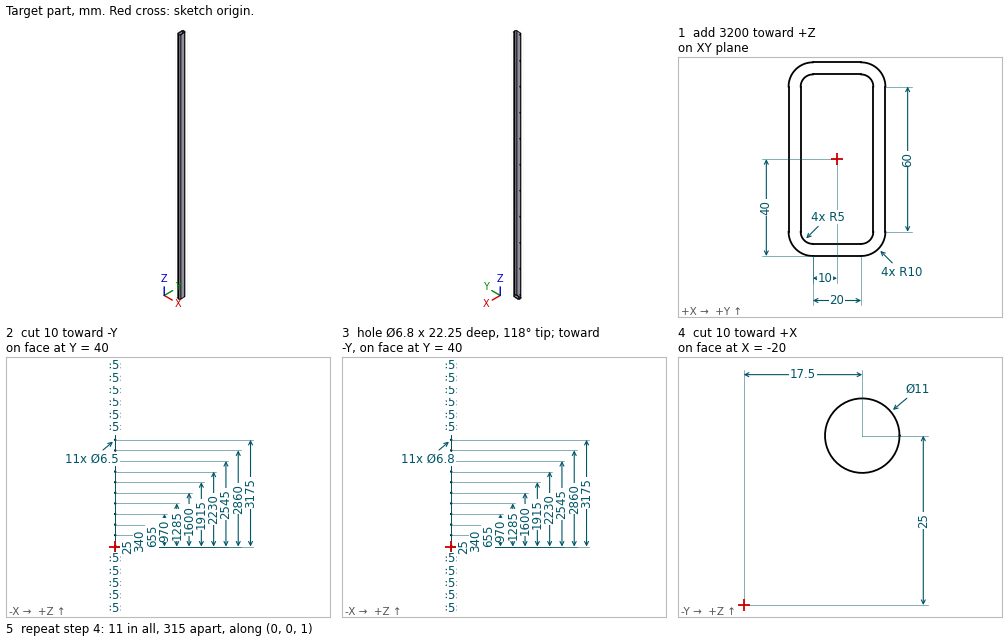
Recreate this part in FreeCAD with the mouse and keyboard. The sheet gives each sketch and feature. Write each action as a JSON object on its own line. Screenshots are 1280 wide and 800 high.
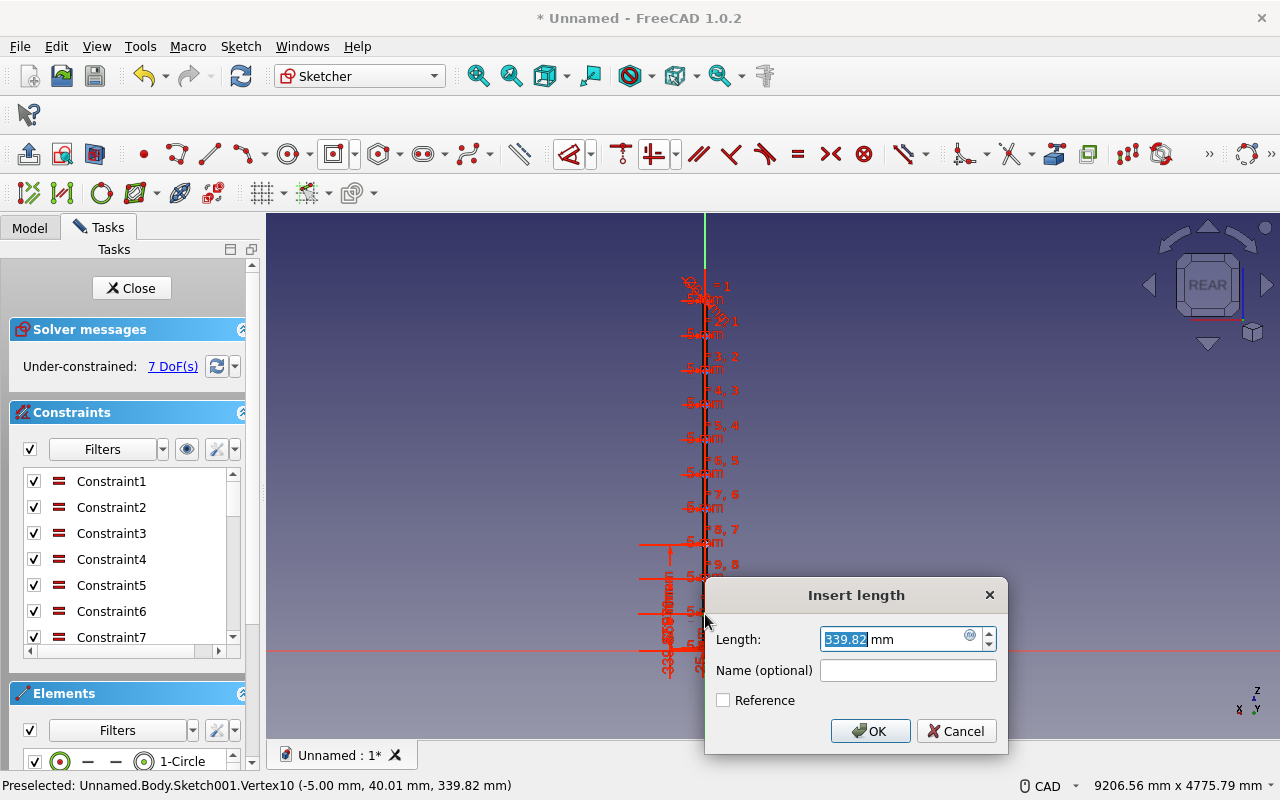
{"action": "type", "text": "340"}
{"action": "key", "text": "Return"}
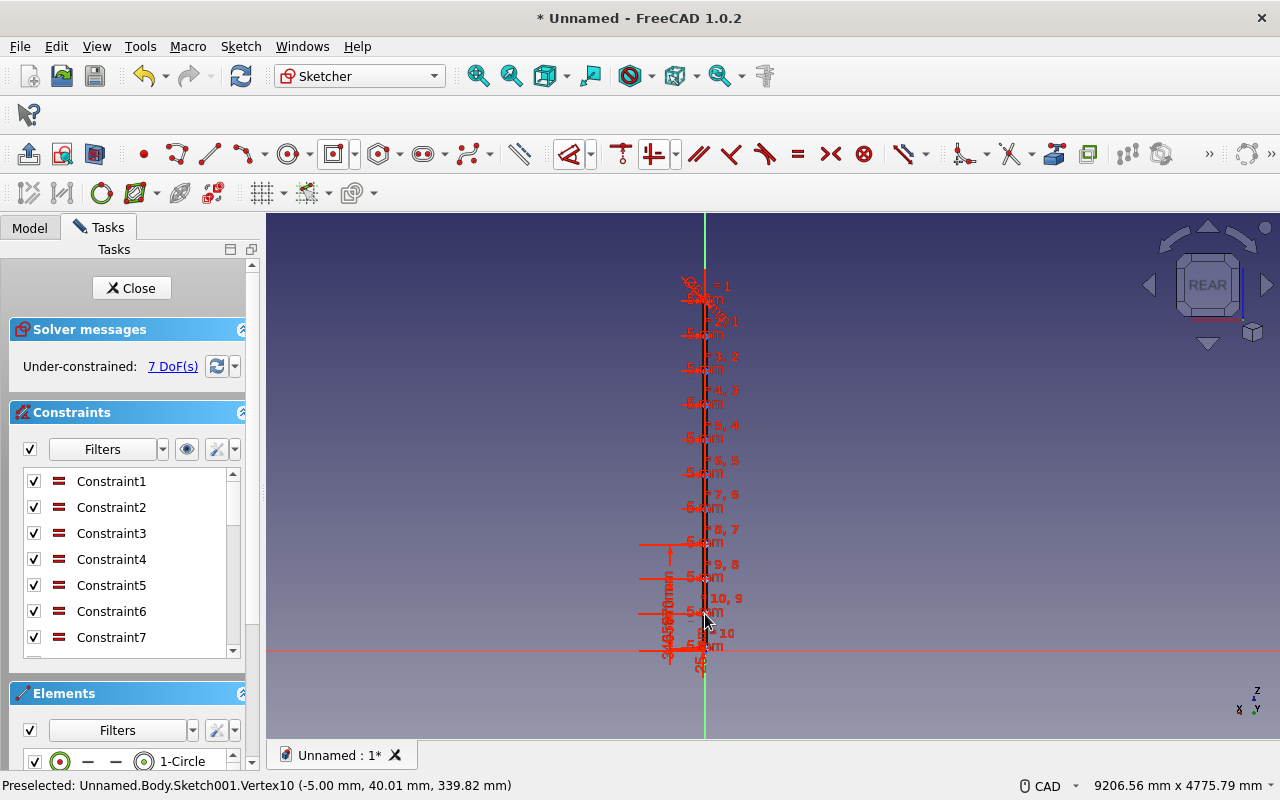
{"action": "left_click", "coordinate": [705, 302]}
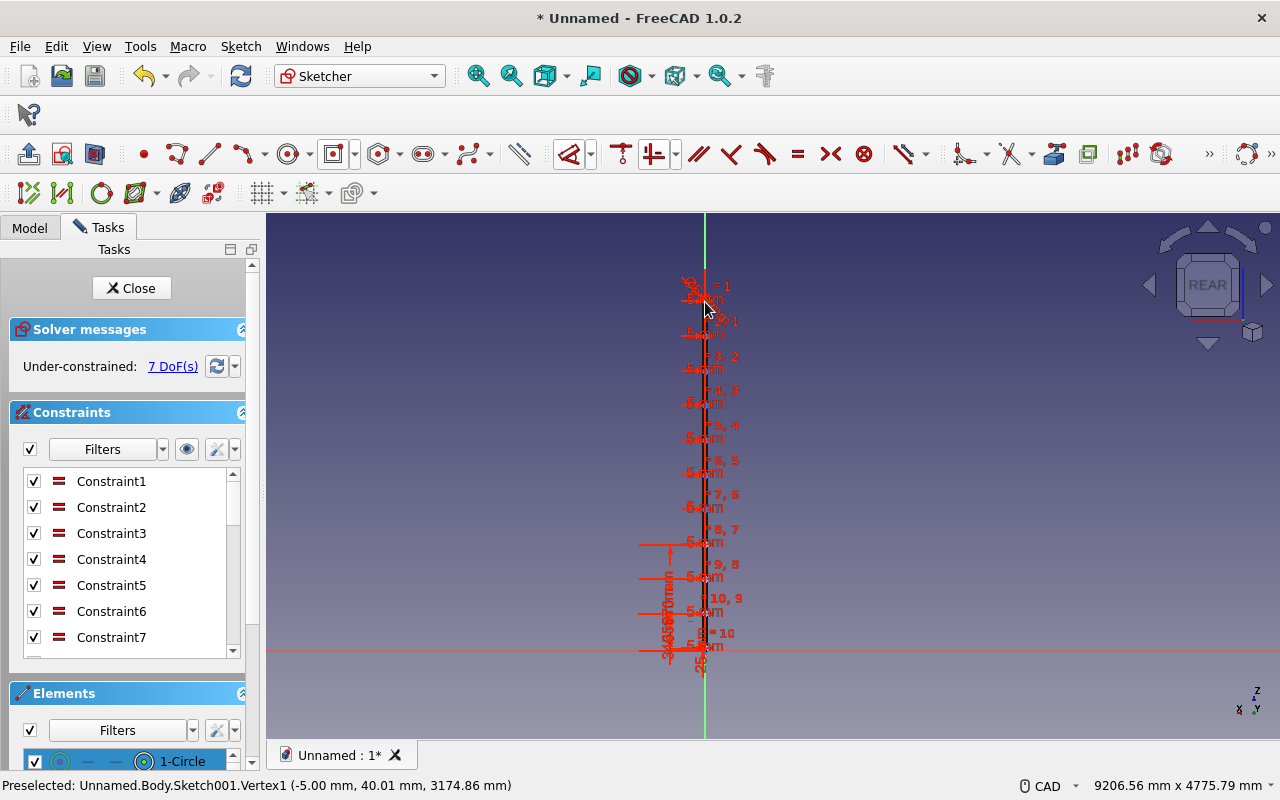
{"action": "left_click", "coordinate": [590, 154]}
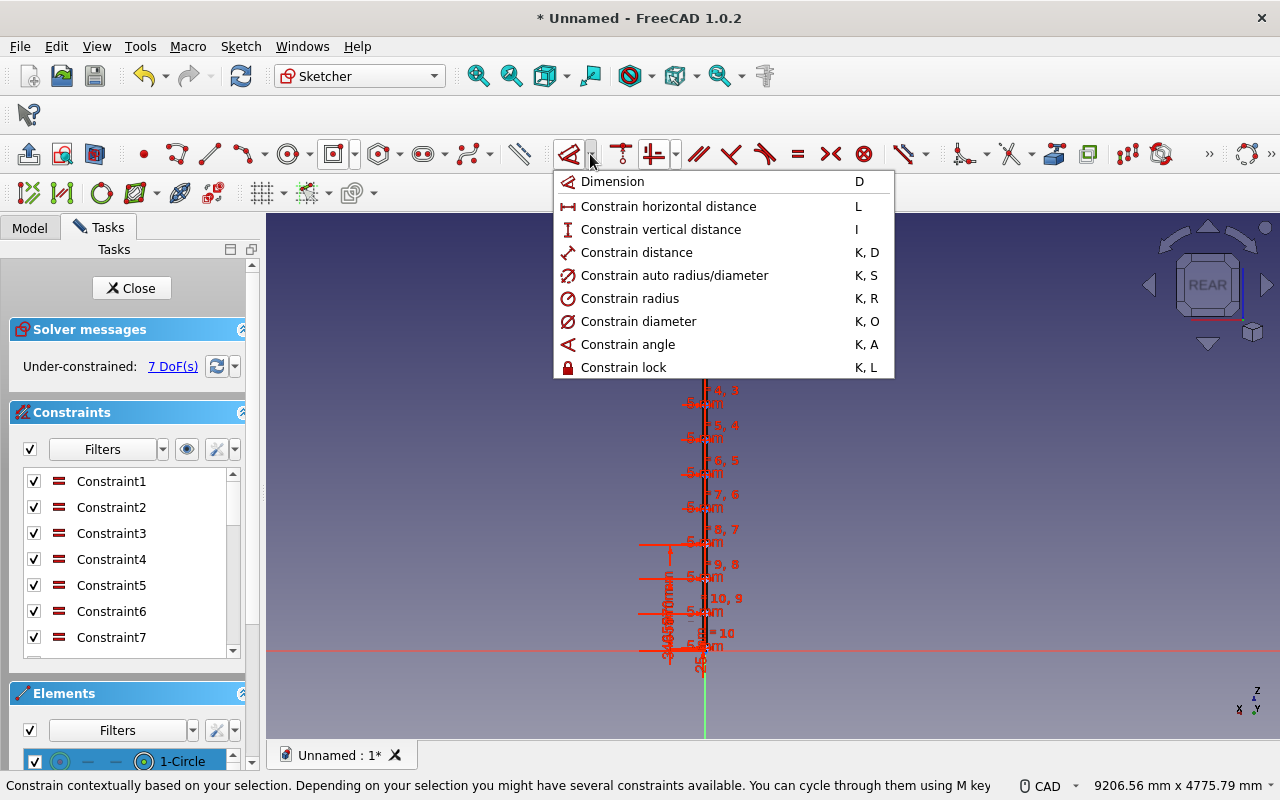
{"action": "left_click", "coordinate": [724, 230]}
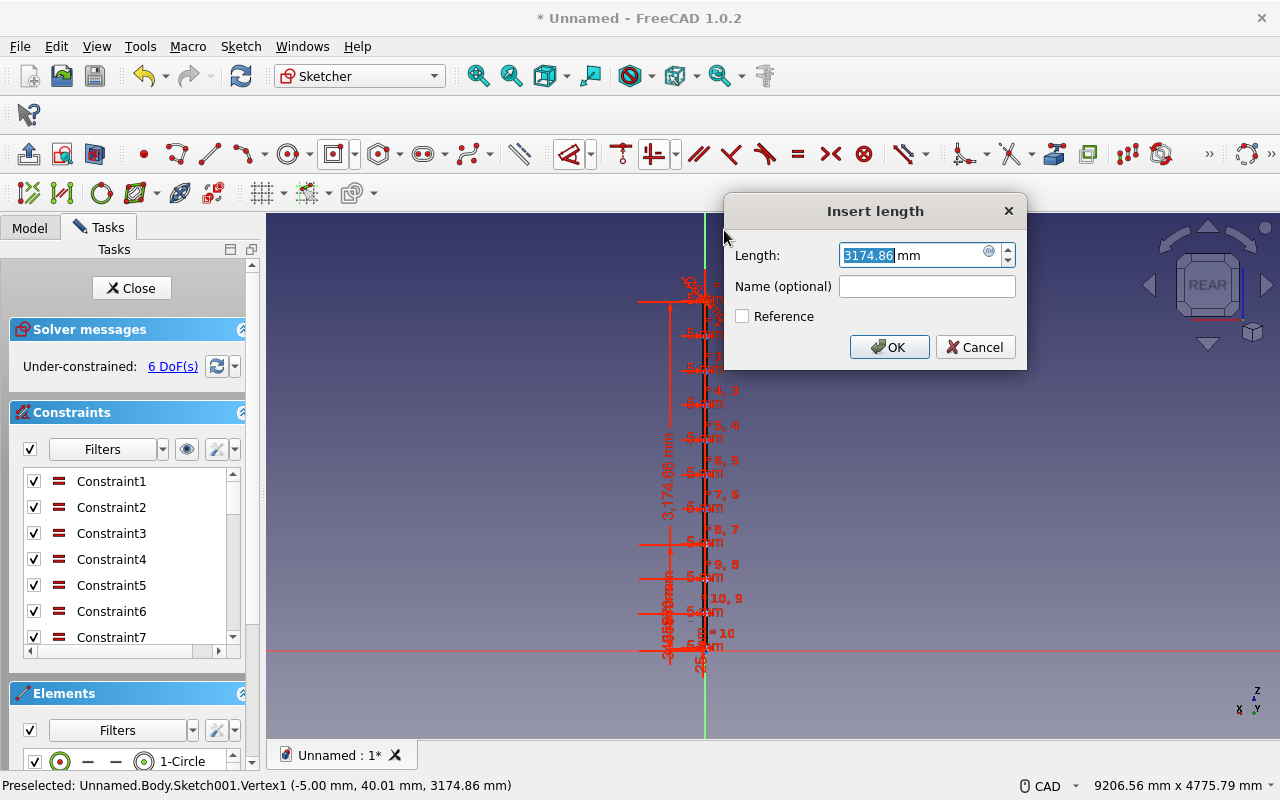
{"action": "type", "text": "3175"}
{"action": "key", "text": "Return"}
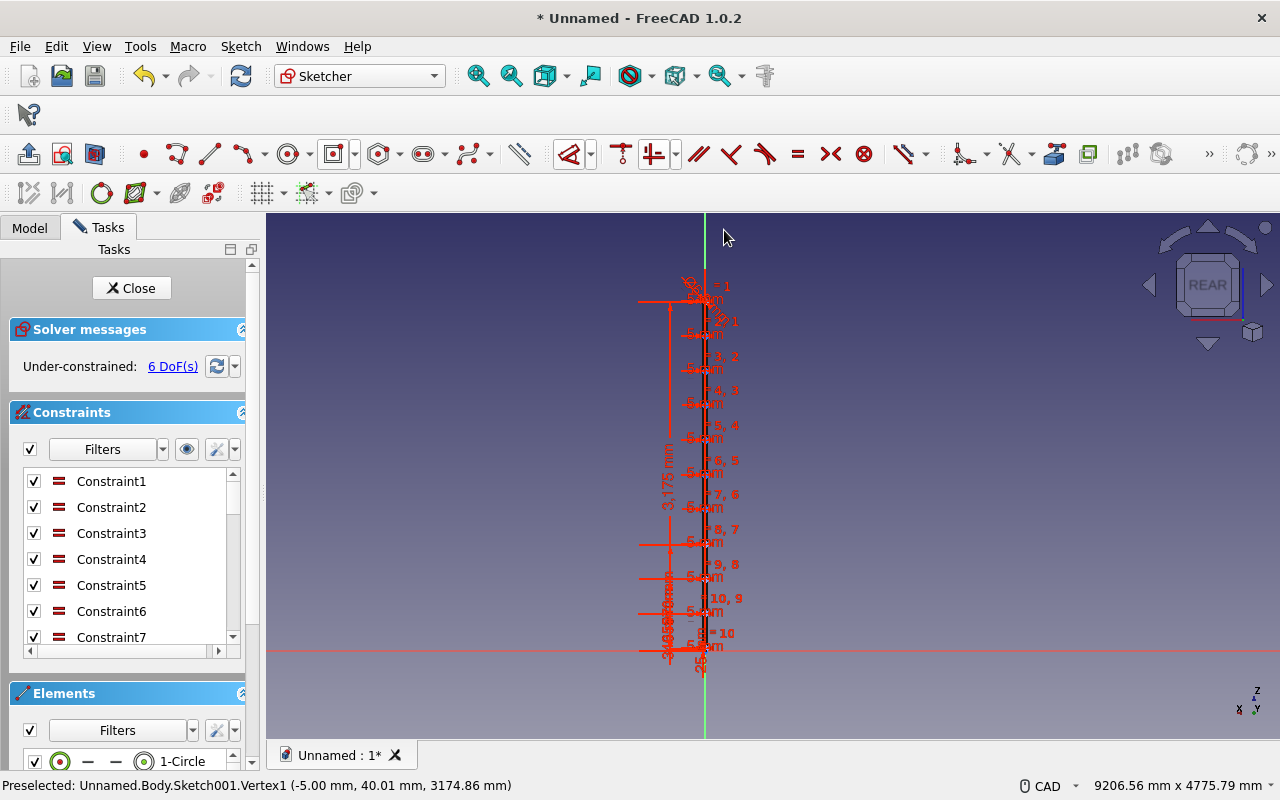
{"action": "left_click", "coordinate": [705, 336]}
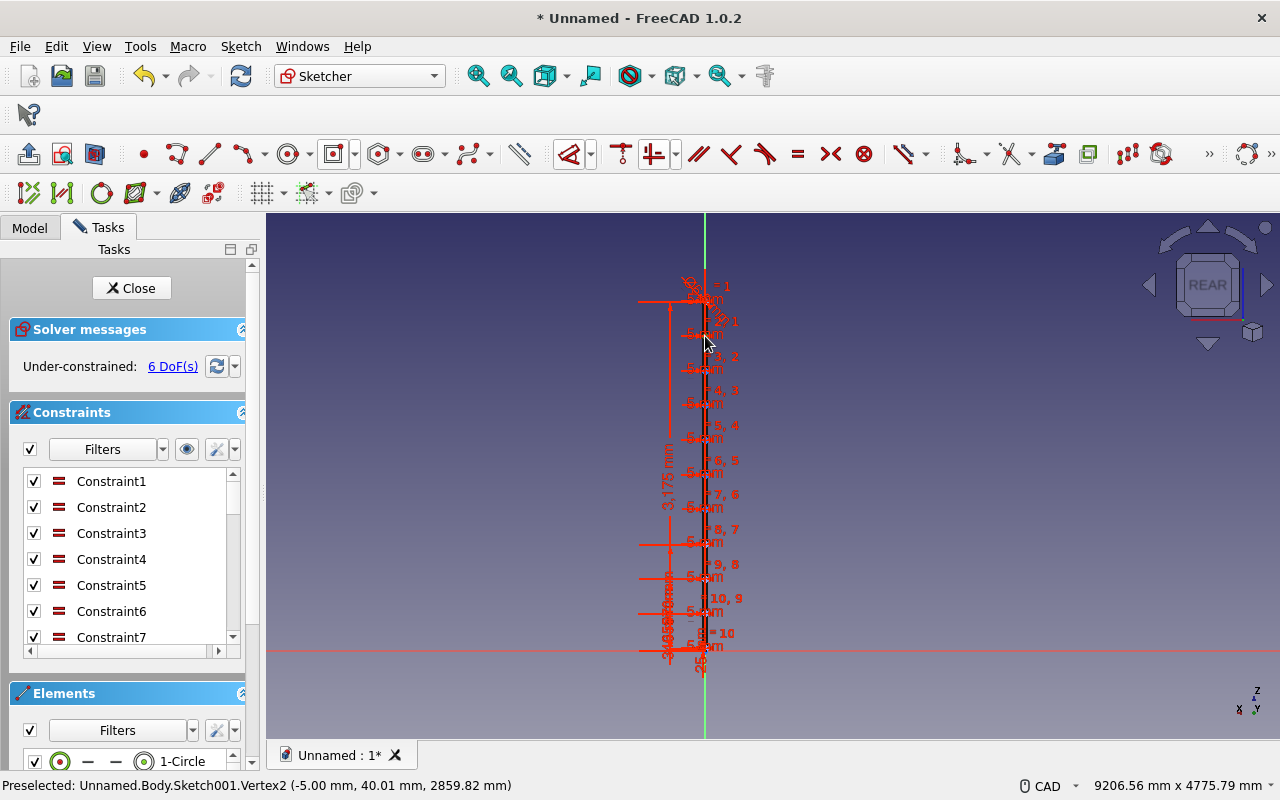
{"action": "left_click", "coordinate": [590, 154]}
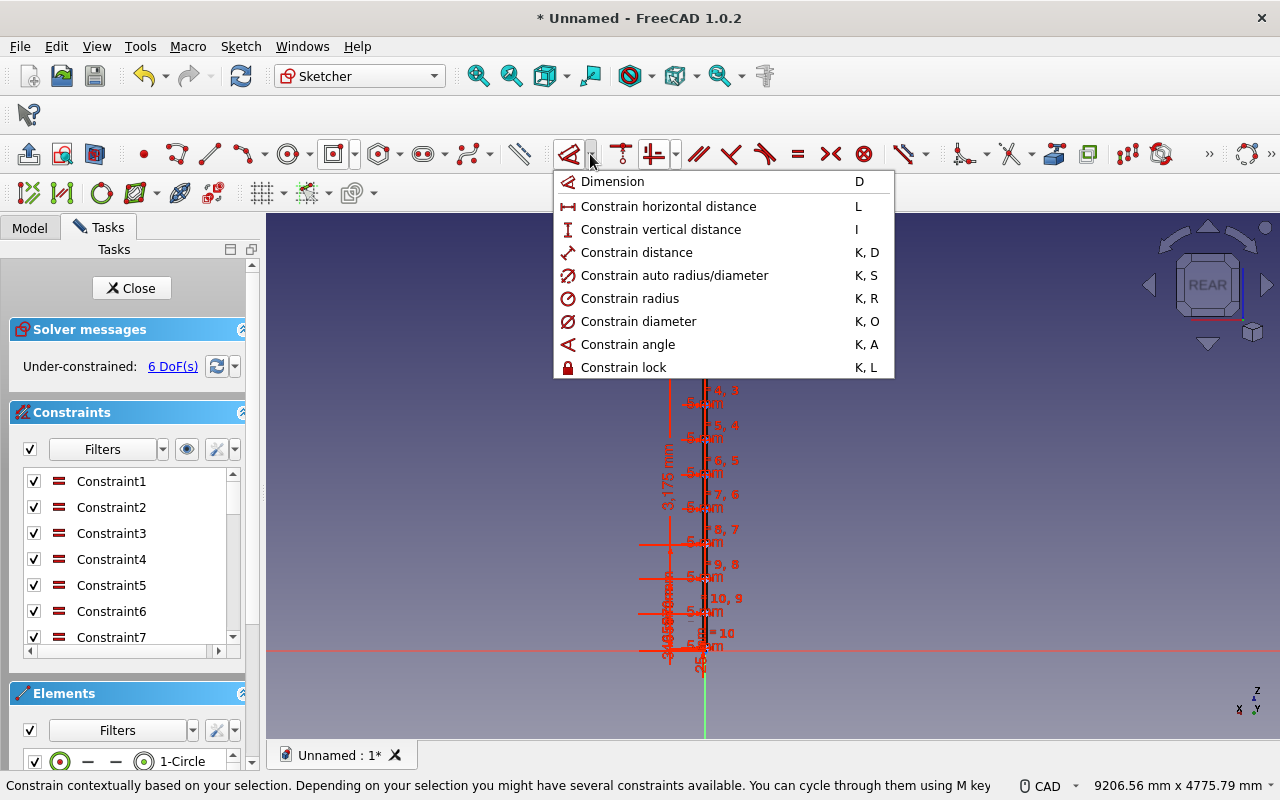
{"action": "left_click", "coordinate": [724, 230]}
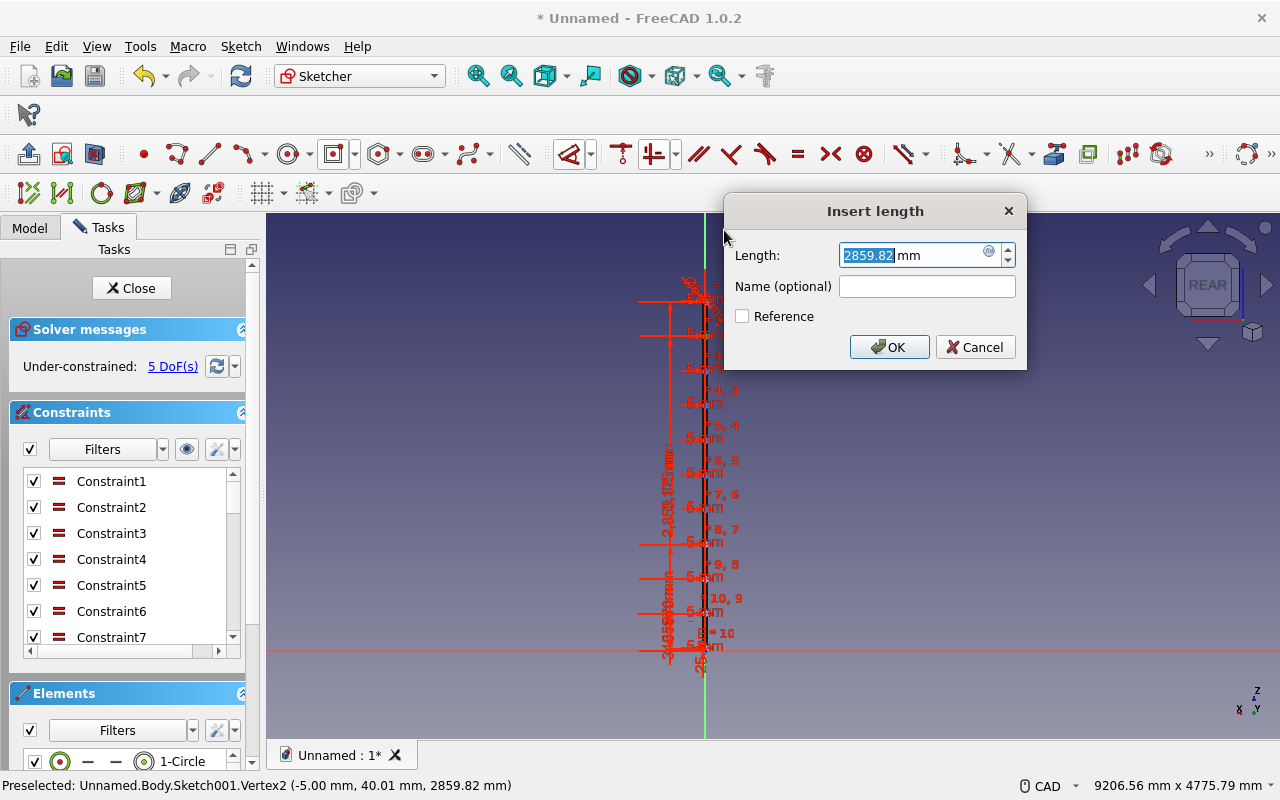
{"action": "type", "text": "2860"}
{"action": "key", "text": "Return"}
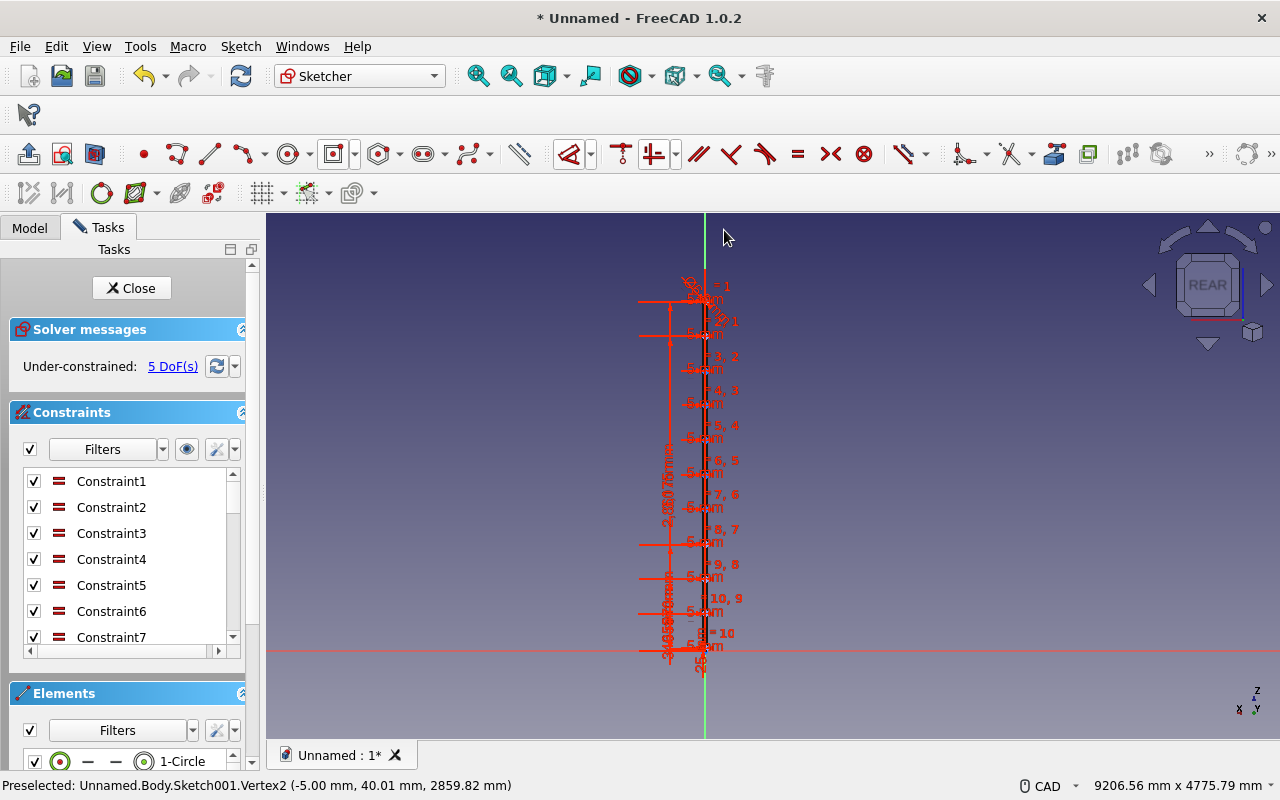
{"action": "left_click", "coordinate": [705, 371]}